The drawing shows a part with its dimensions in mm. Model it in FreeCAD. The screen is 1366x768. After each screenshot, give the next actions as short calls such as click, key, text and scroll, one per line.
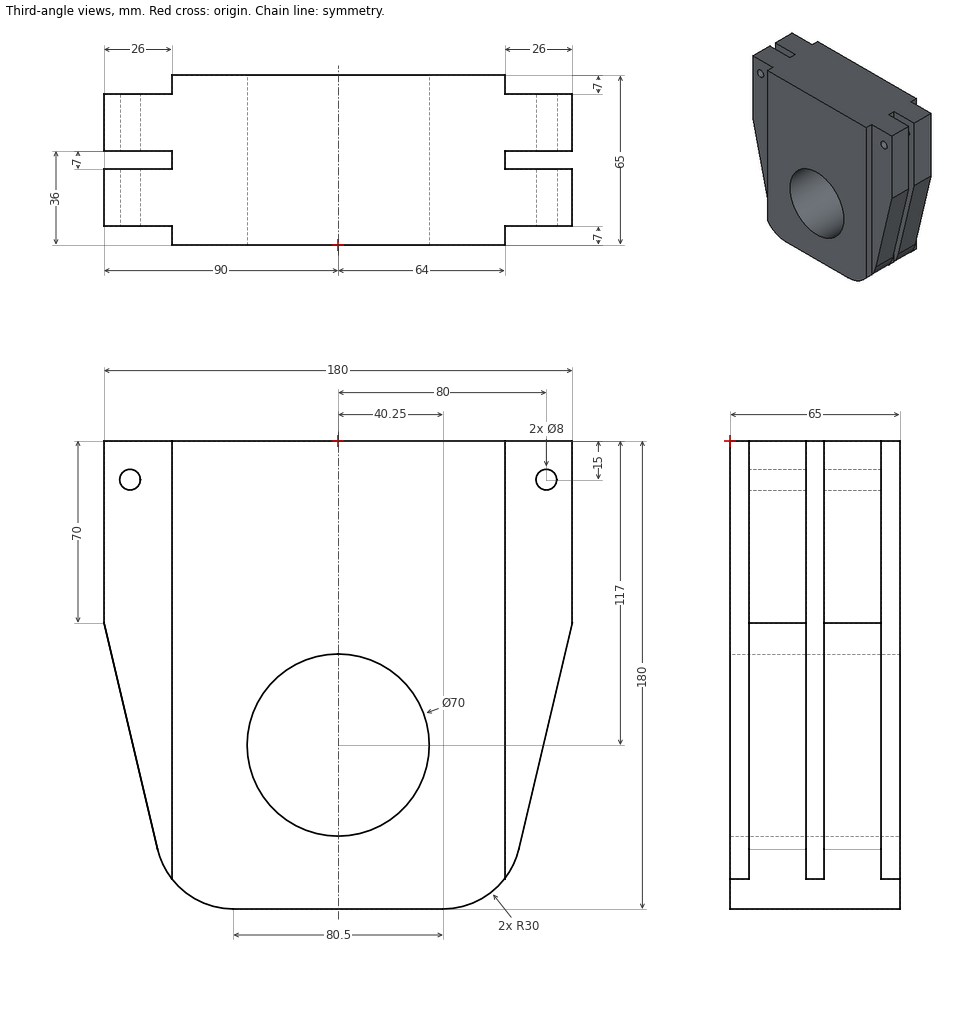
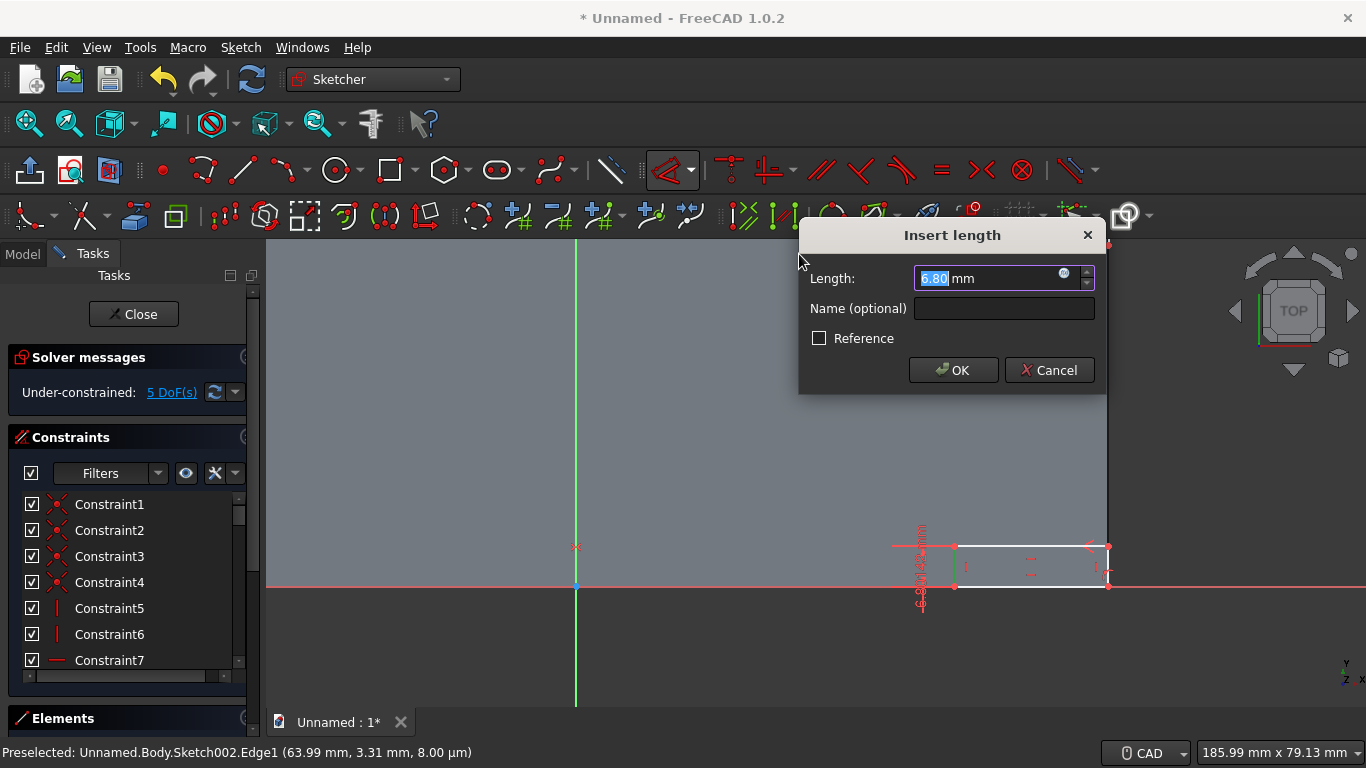
text(7)
key(Return)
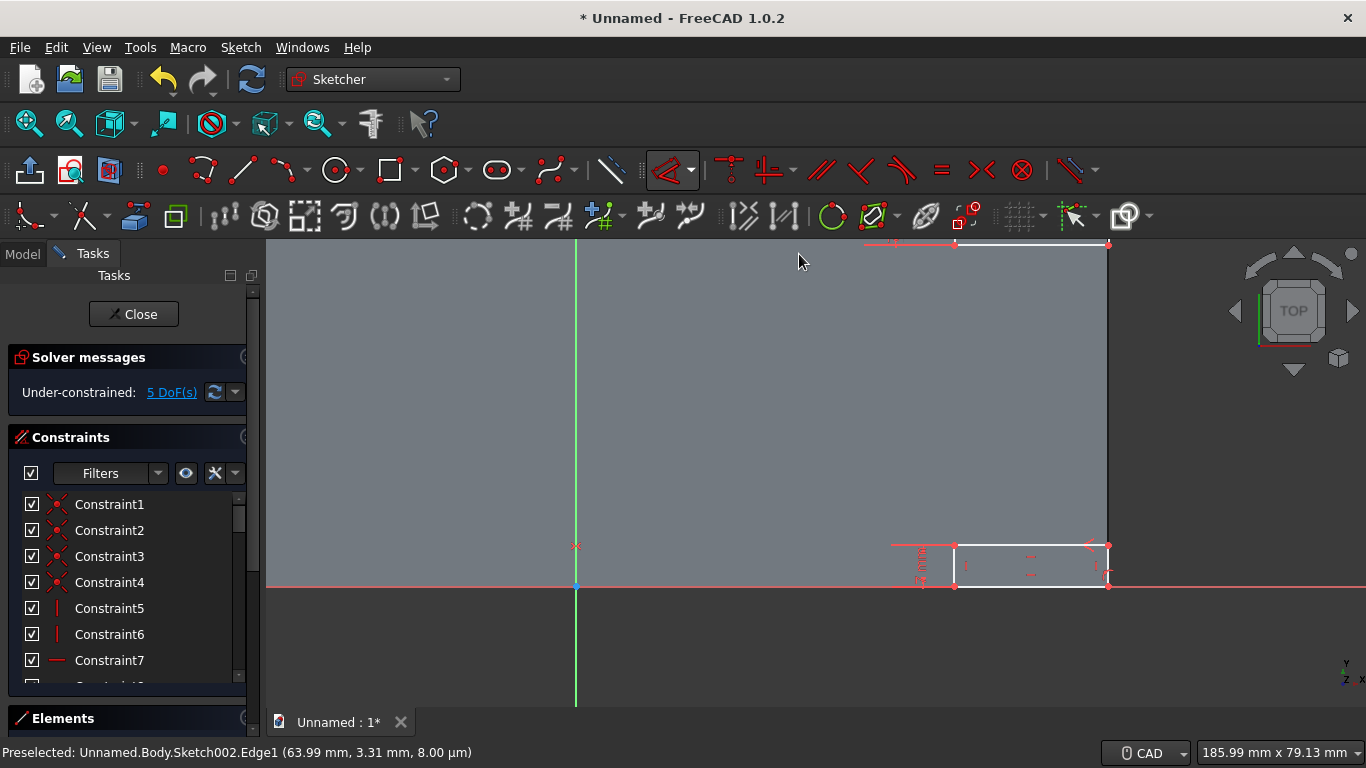
click(1001, 587)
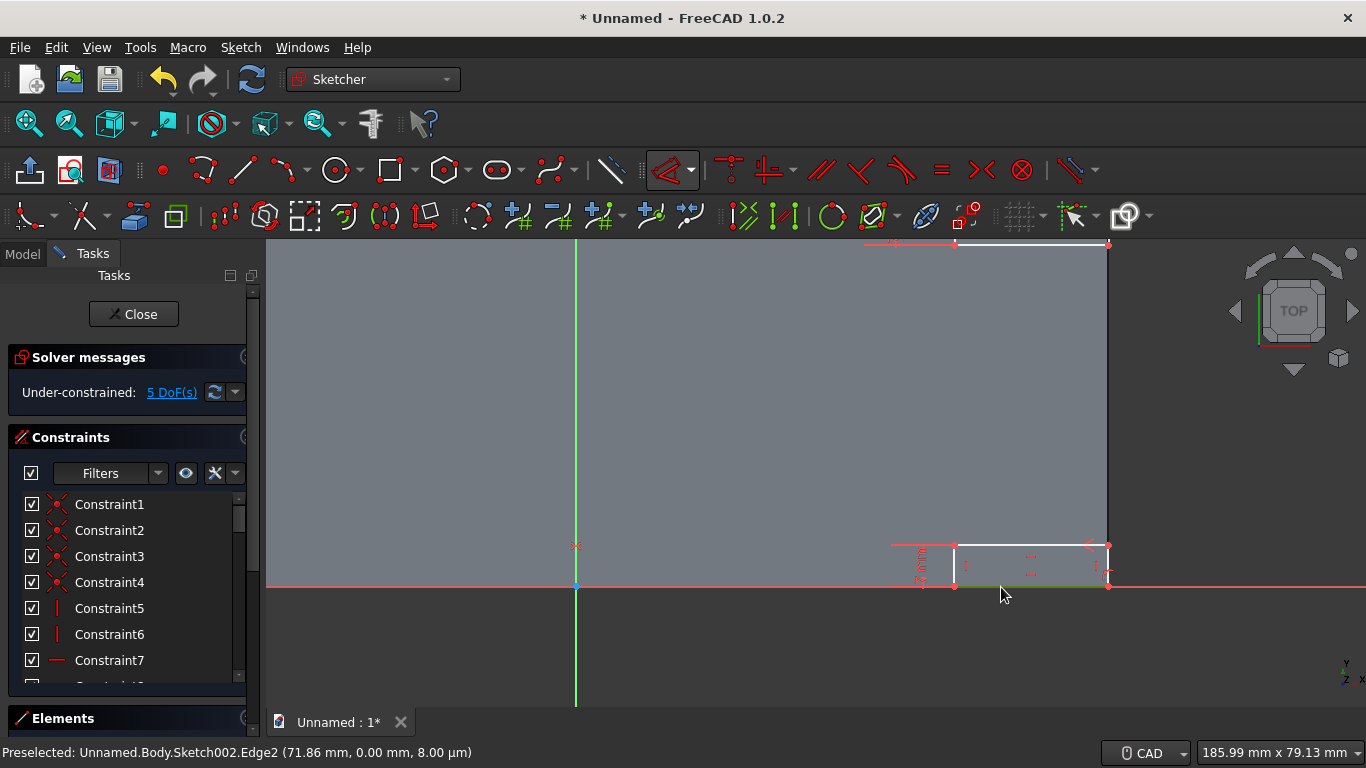
key(l)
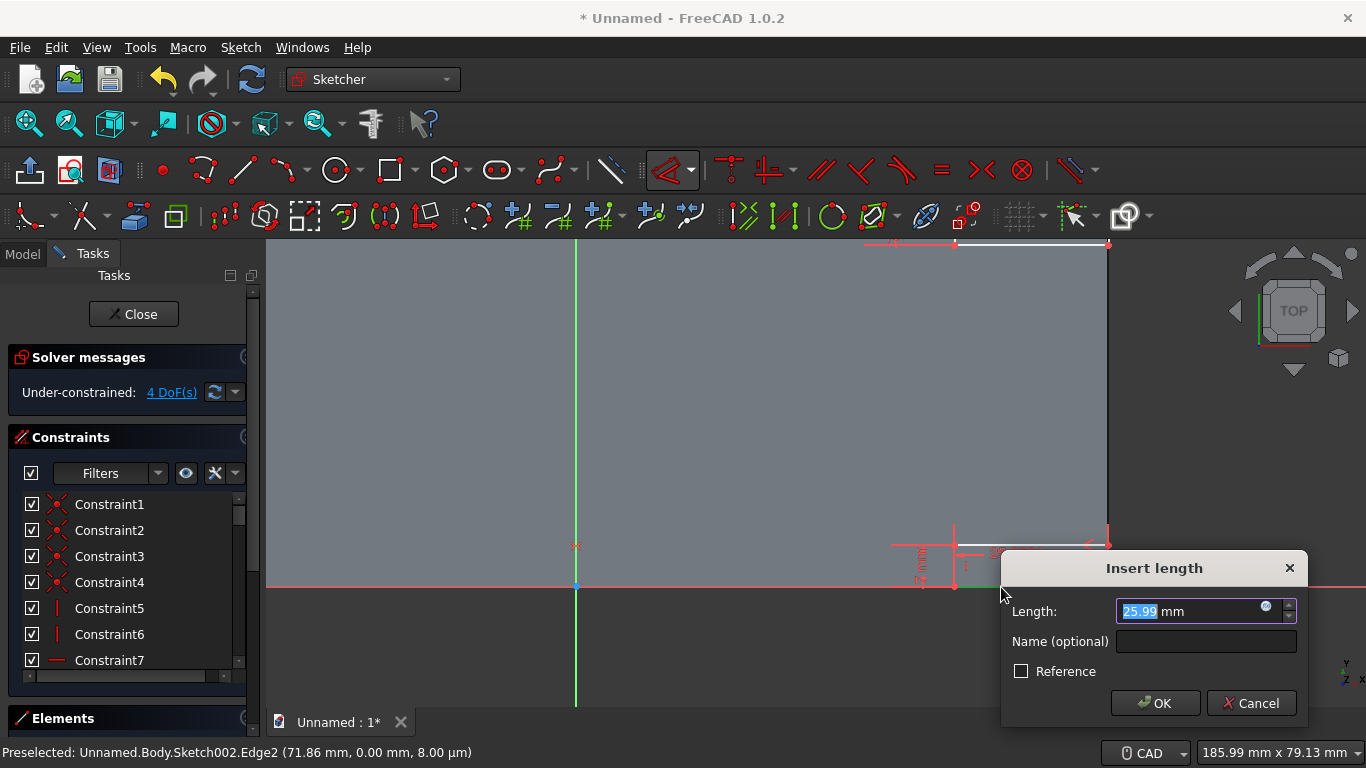
text(26)
key(Return)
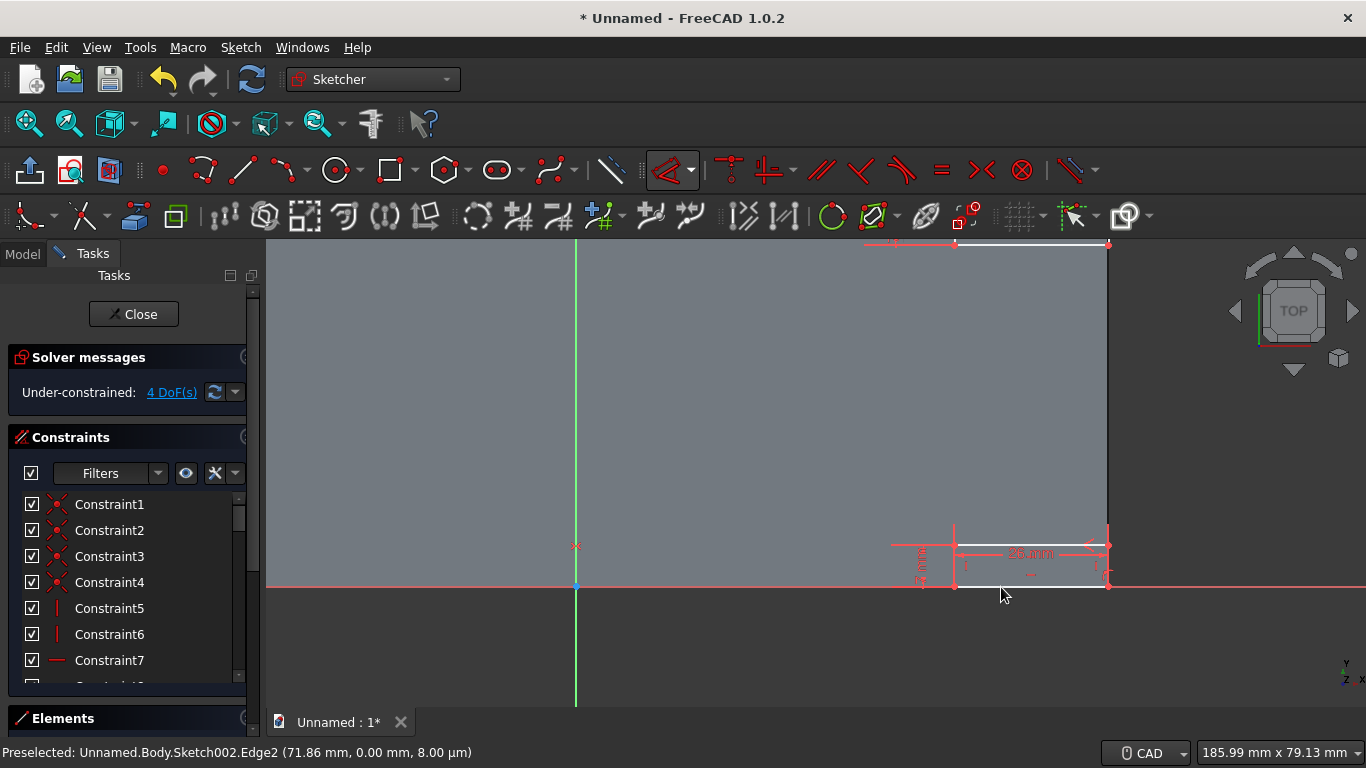
scroll(956, 569, down, 3)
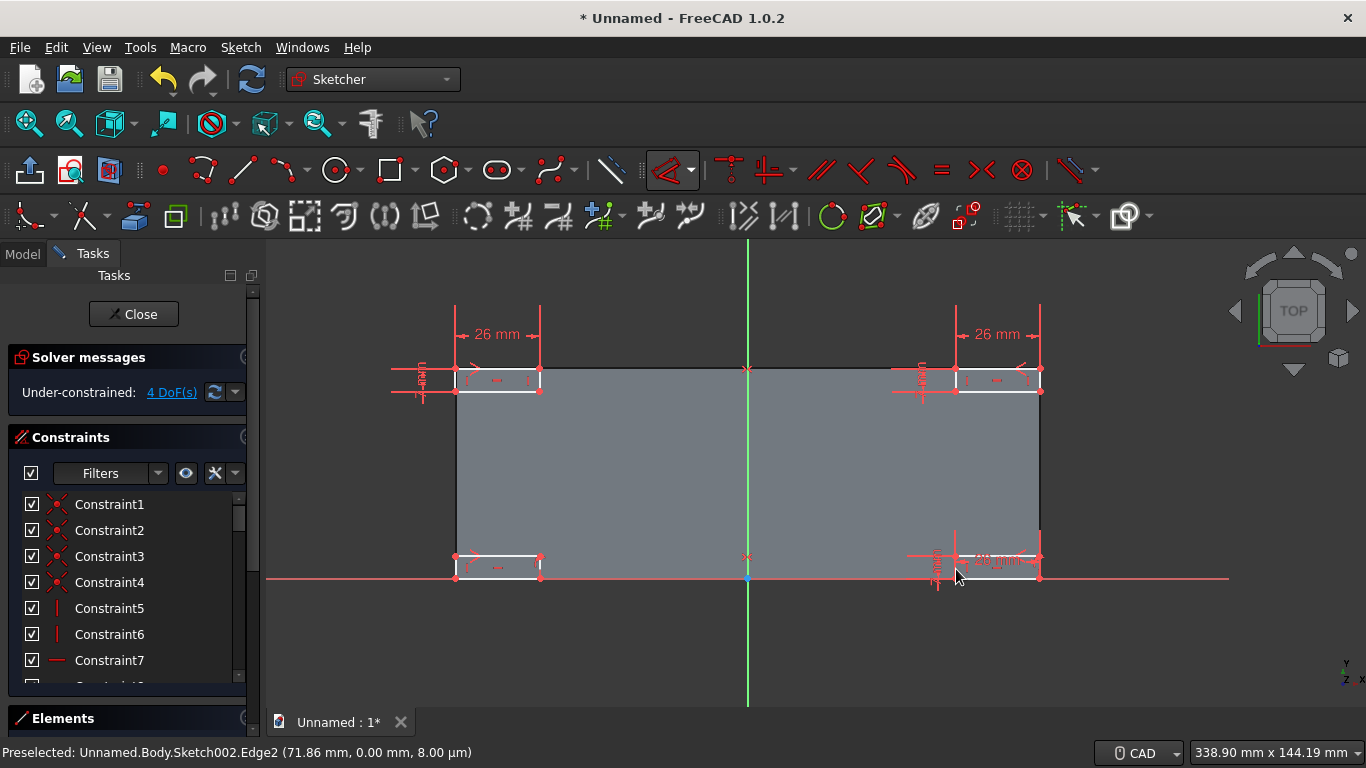
click(481, 579)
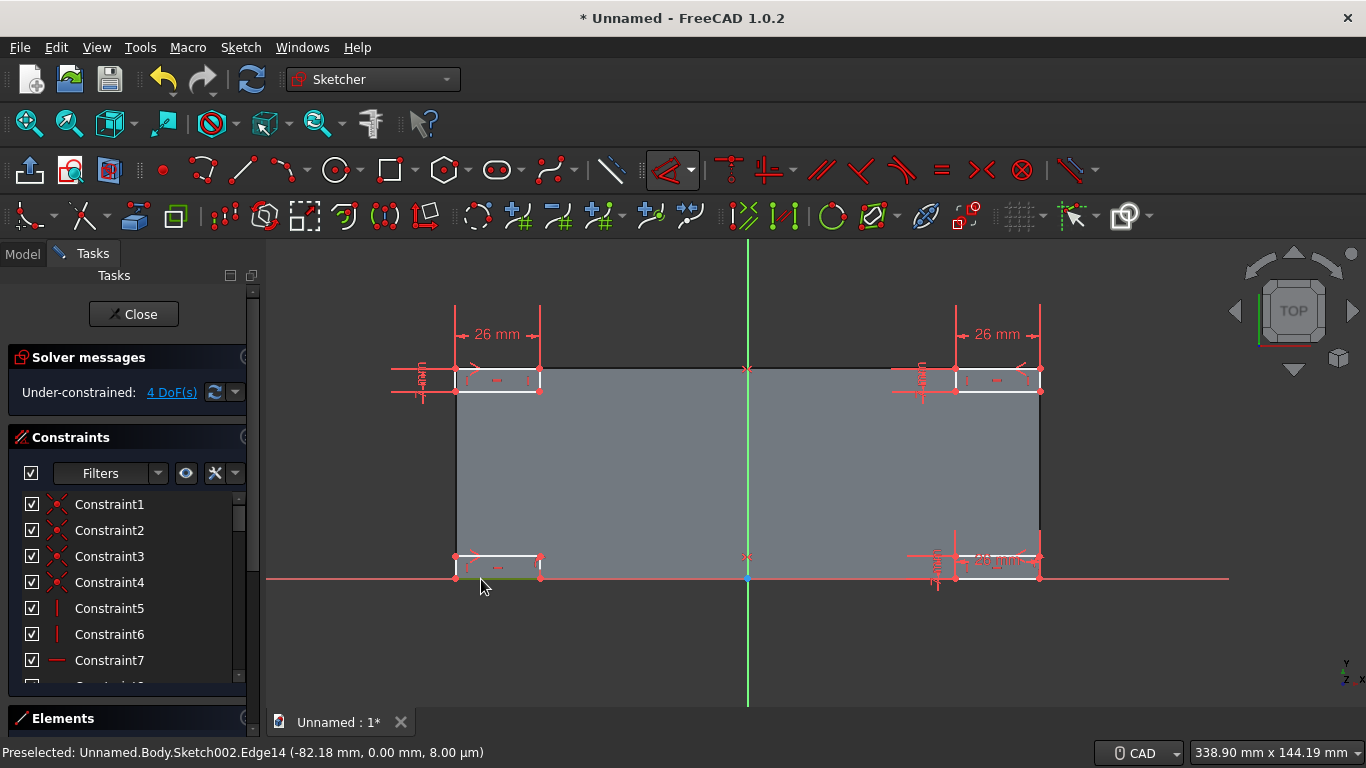
key(l)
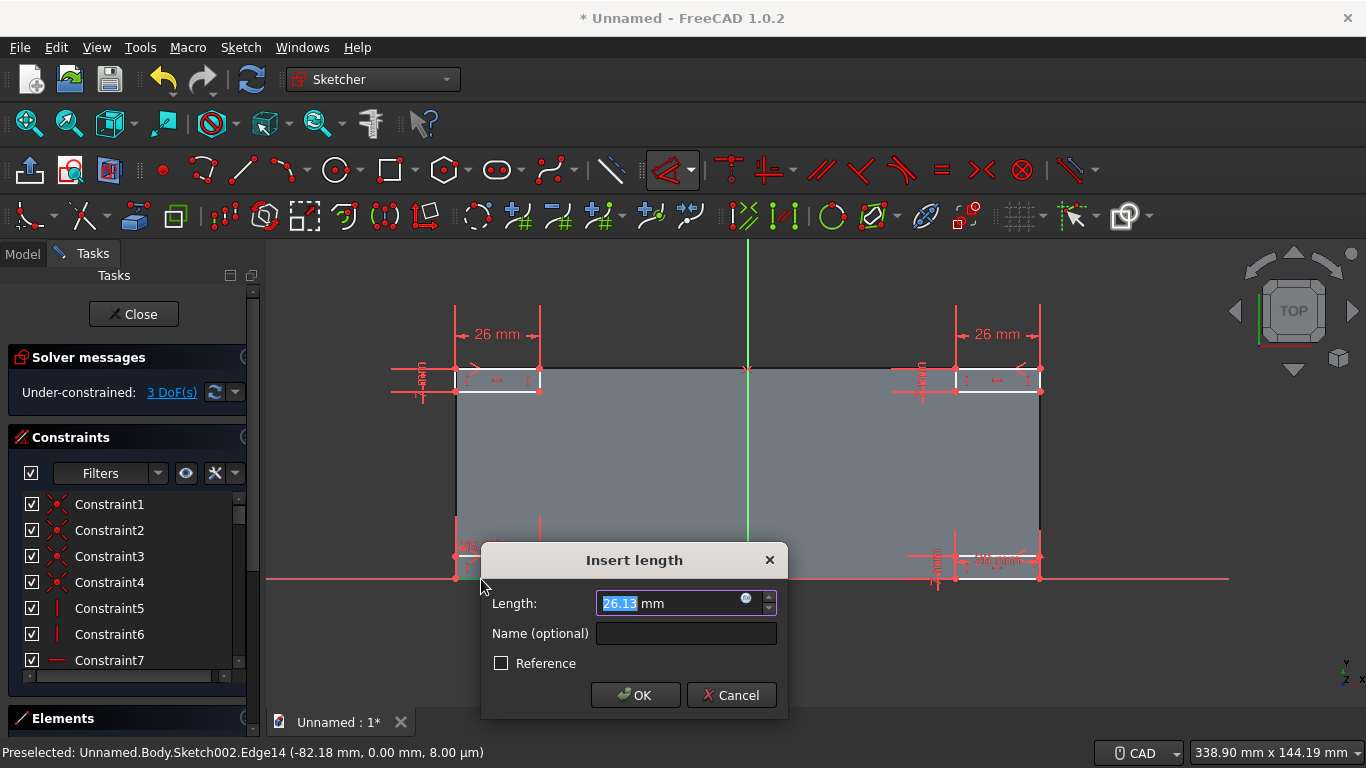
text(26)
key(Return)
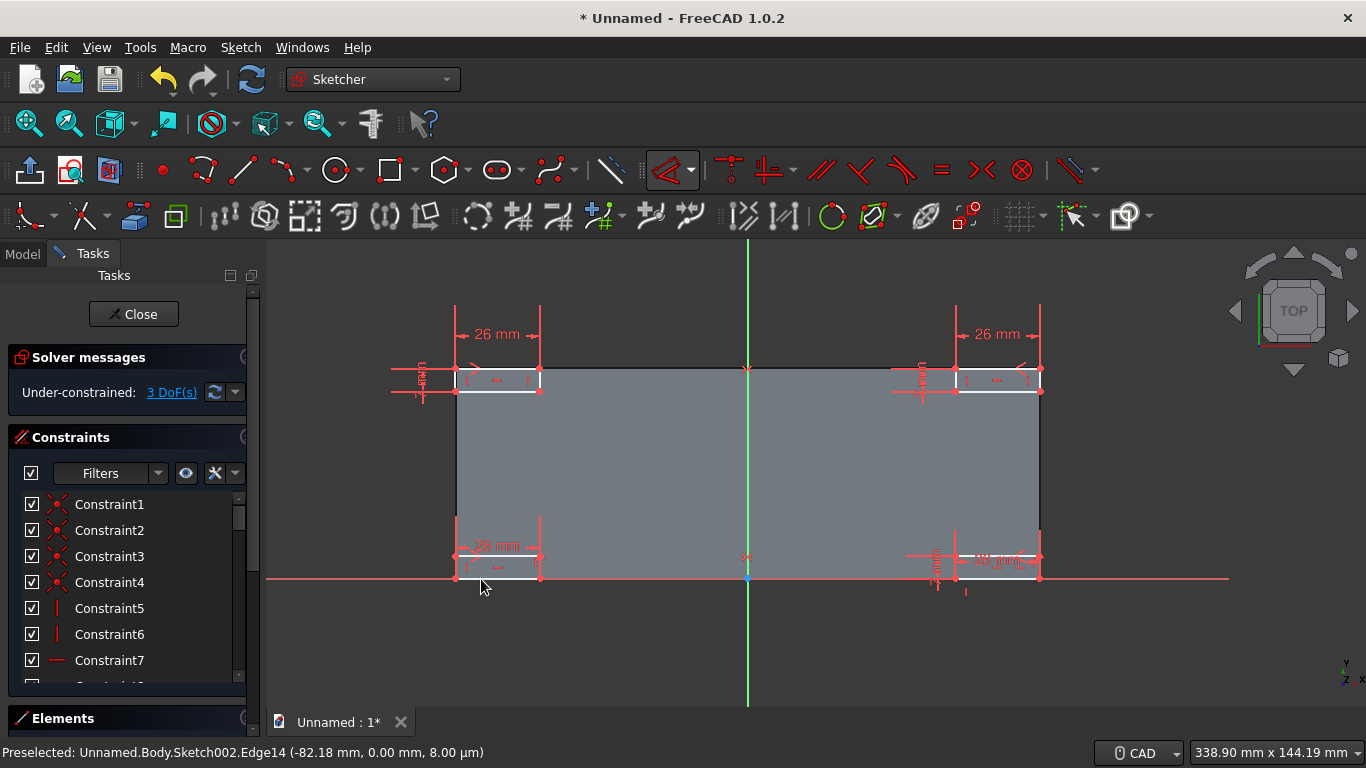
click(955, 556)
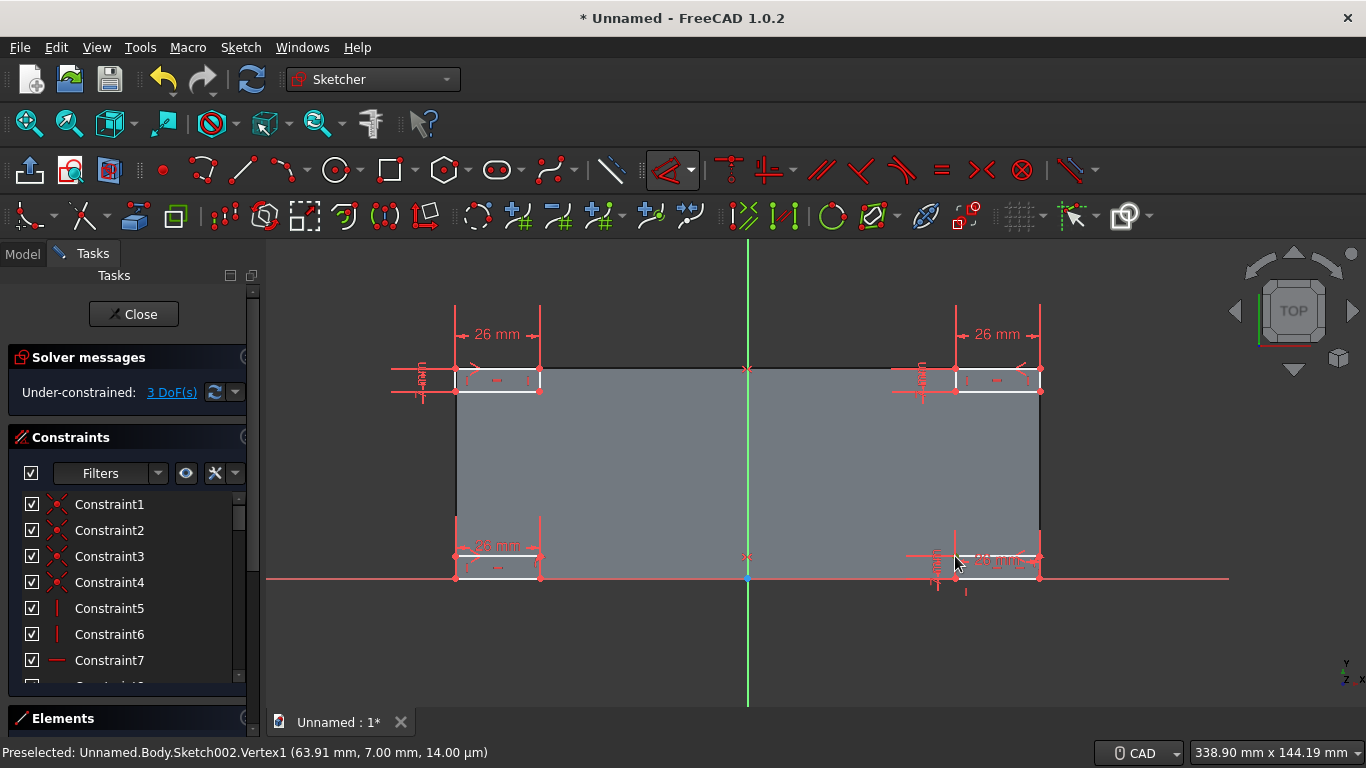
click(694, 170)